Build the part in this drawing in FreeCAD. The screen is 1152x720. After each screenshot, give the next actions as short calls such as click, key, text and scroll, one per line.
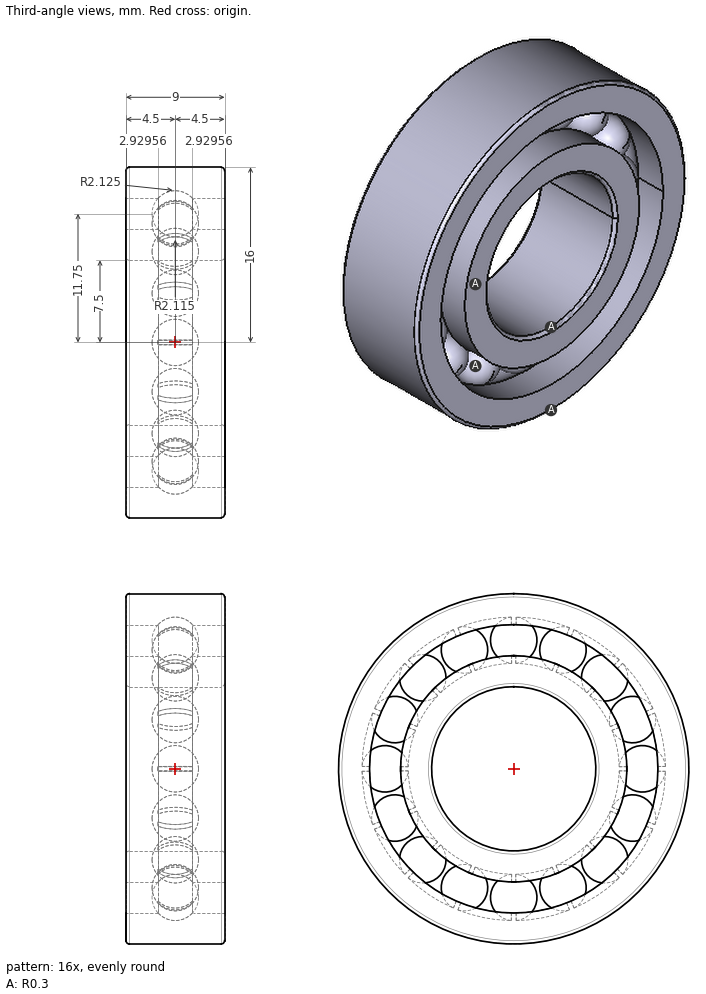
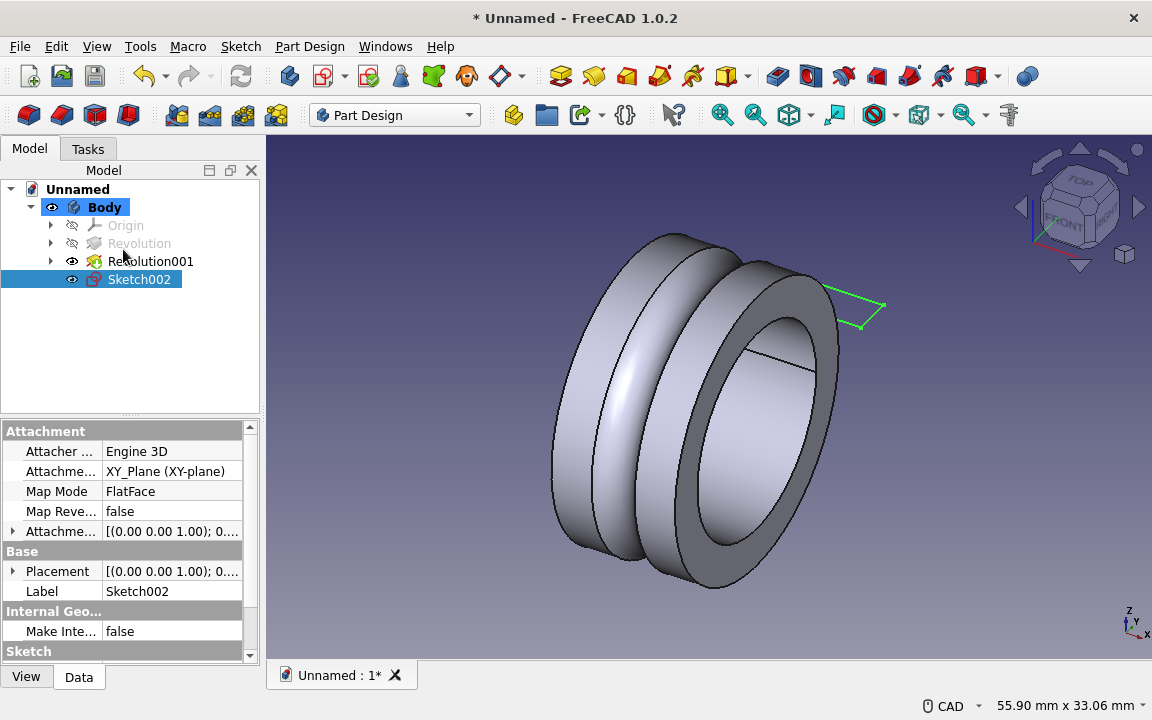
click(594, 76)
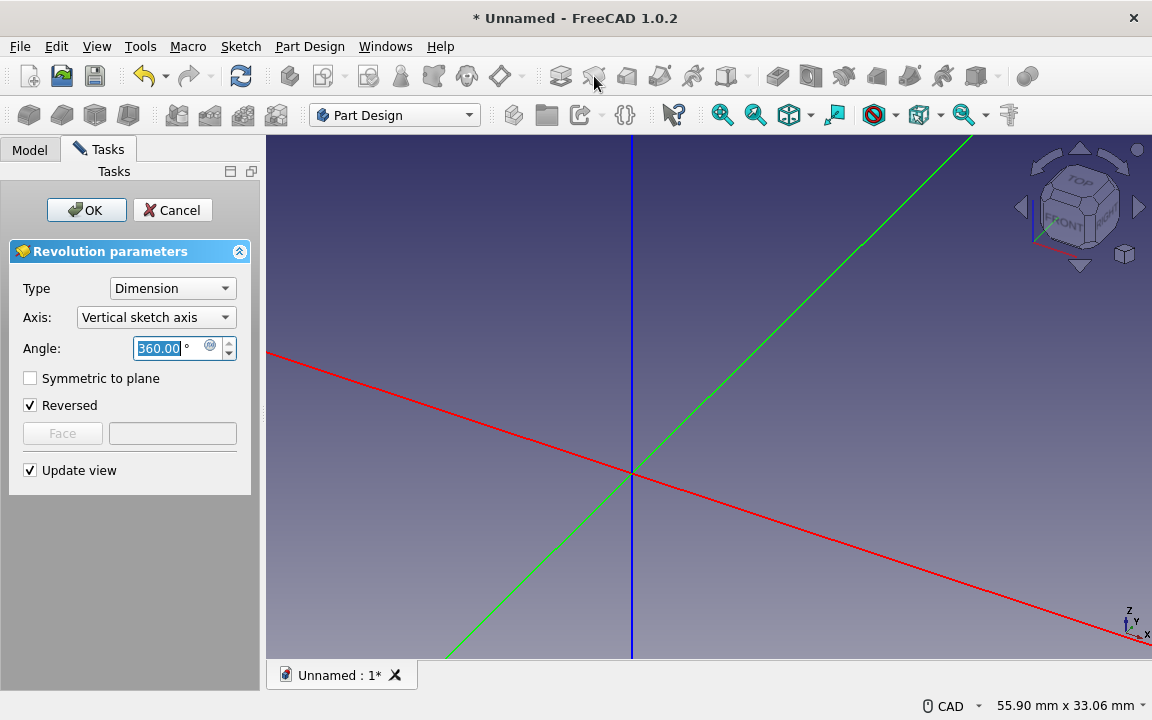
click(157, 318)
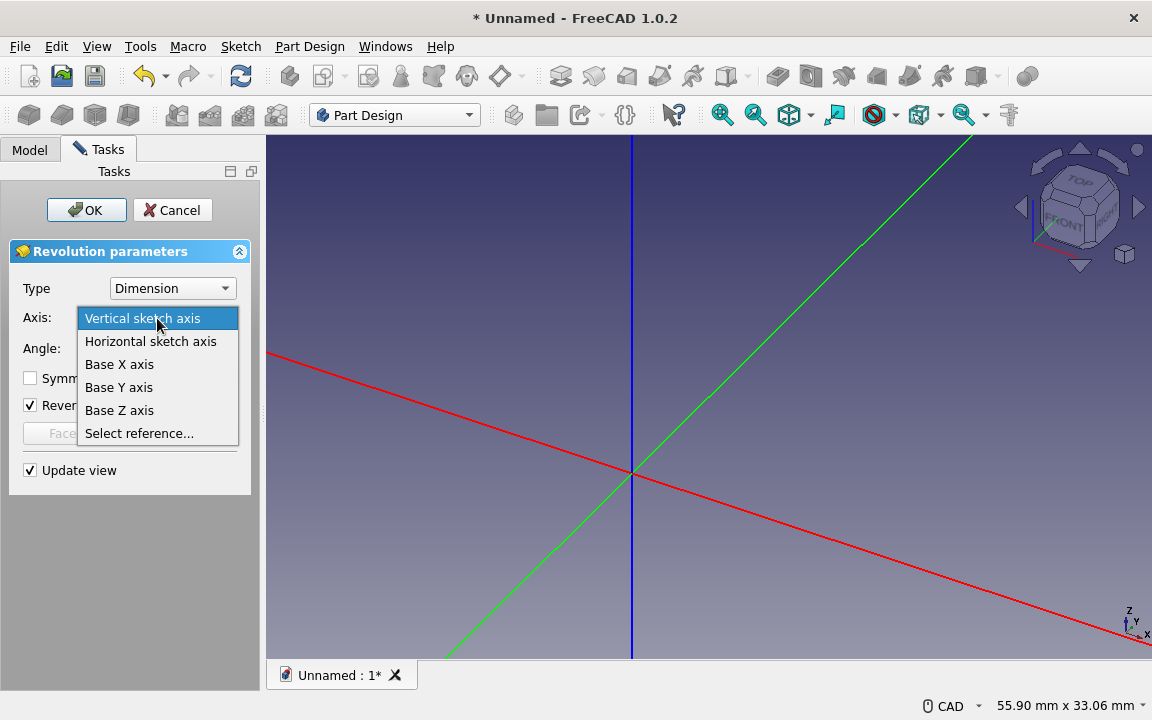
click(156, 342)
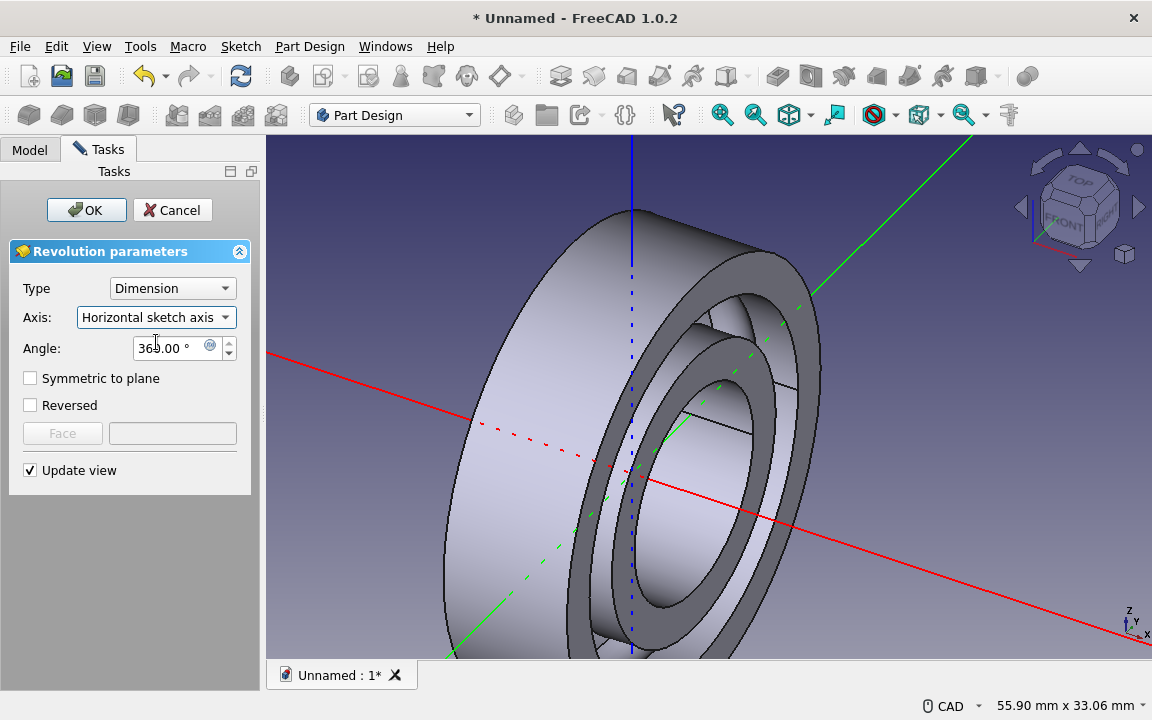
click(87, 210)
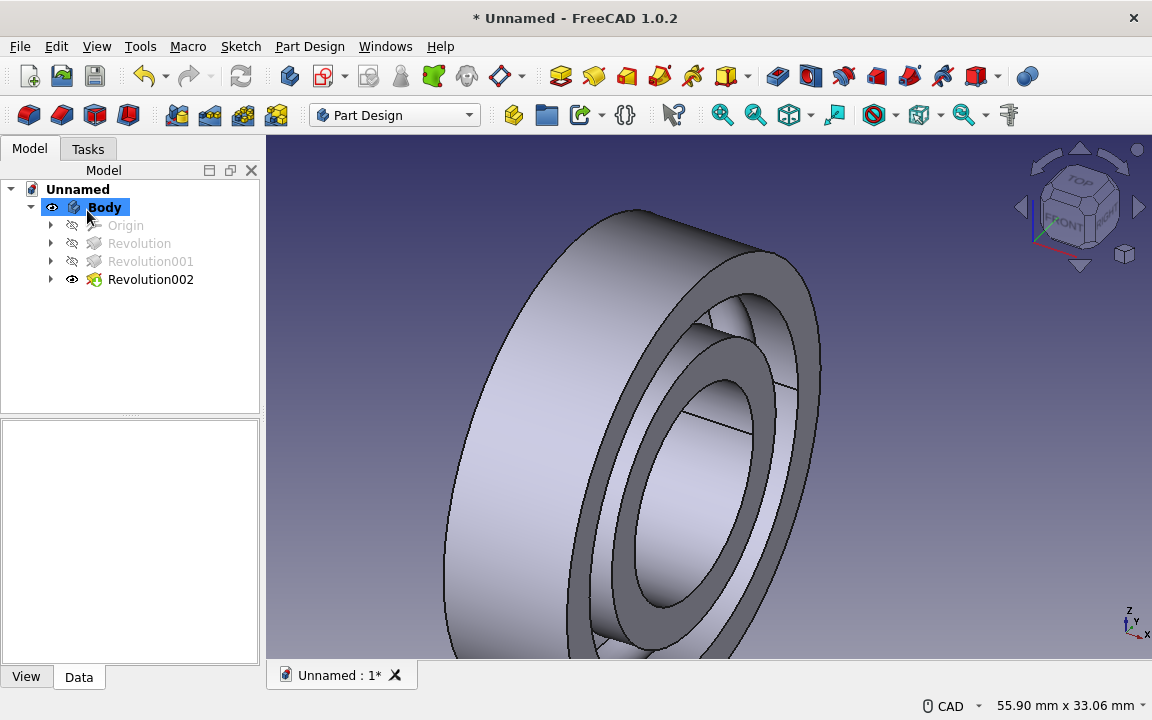
click(723, 116)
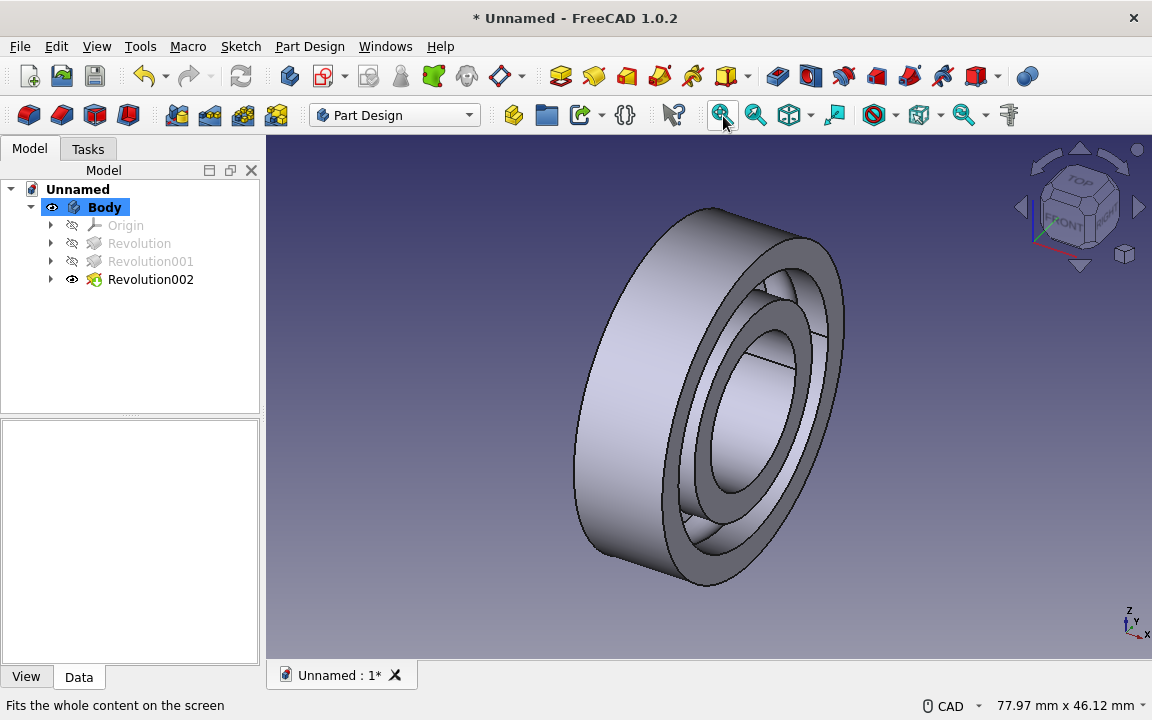
click(117, 243)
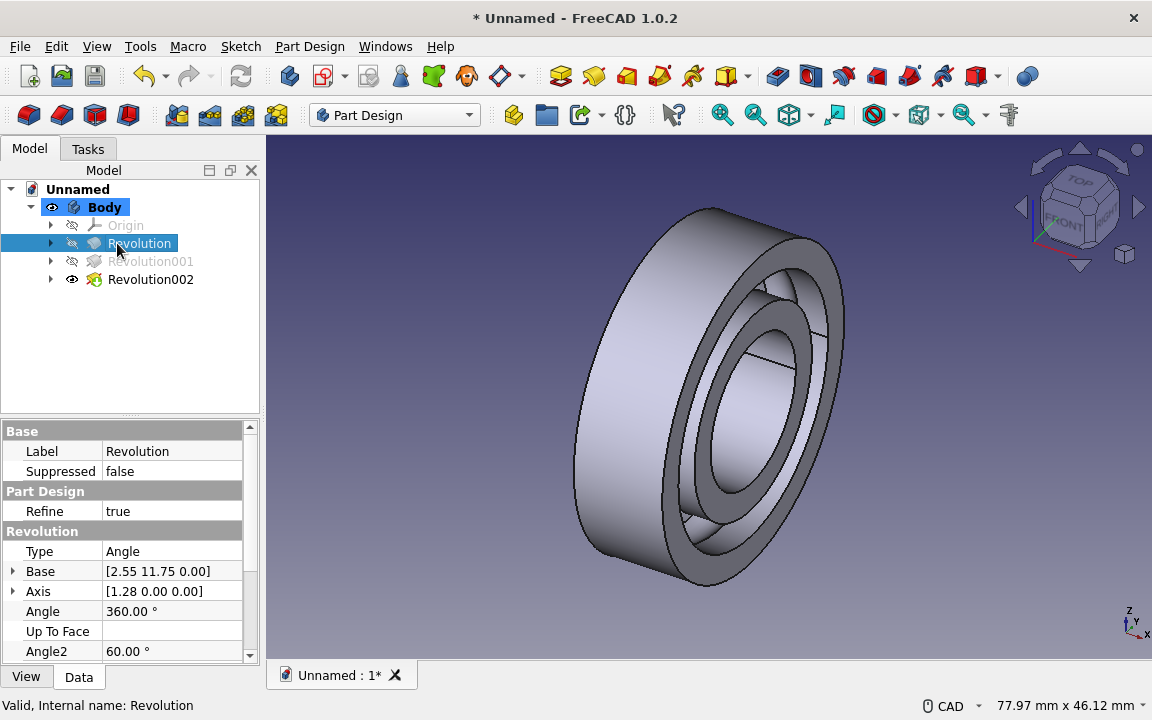
click(243, 116)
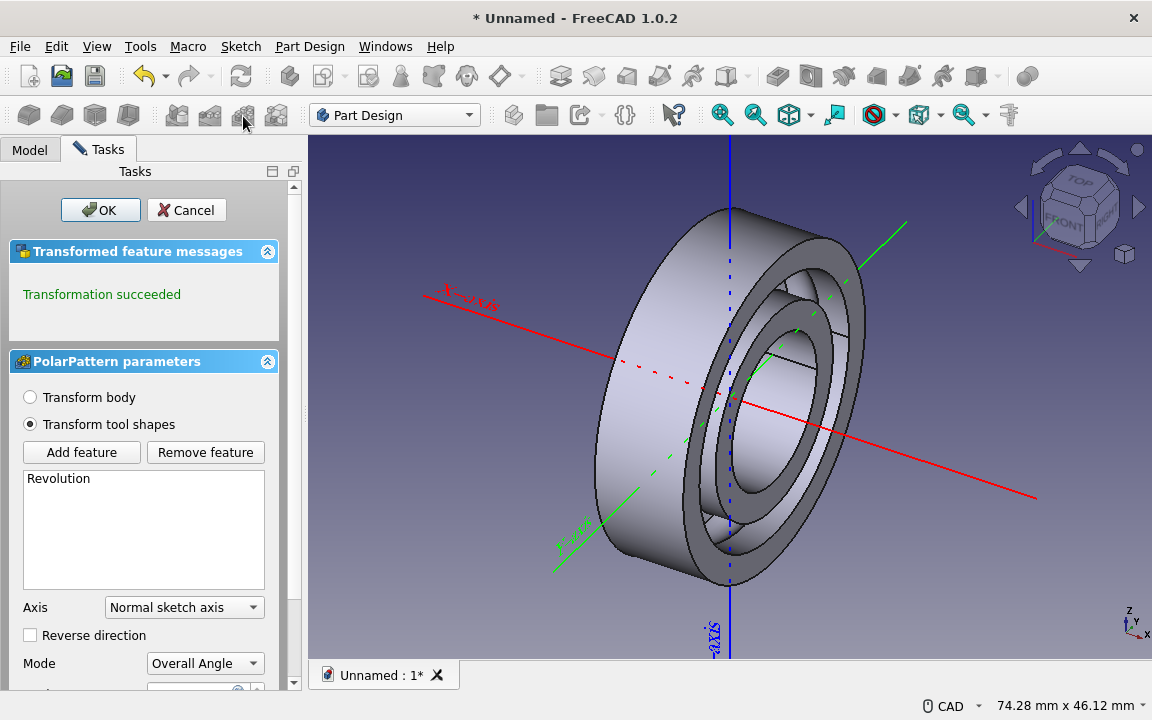
click(185, 608)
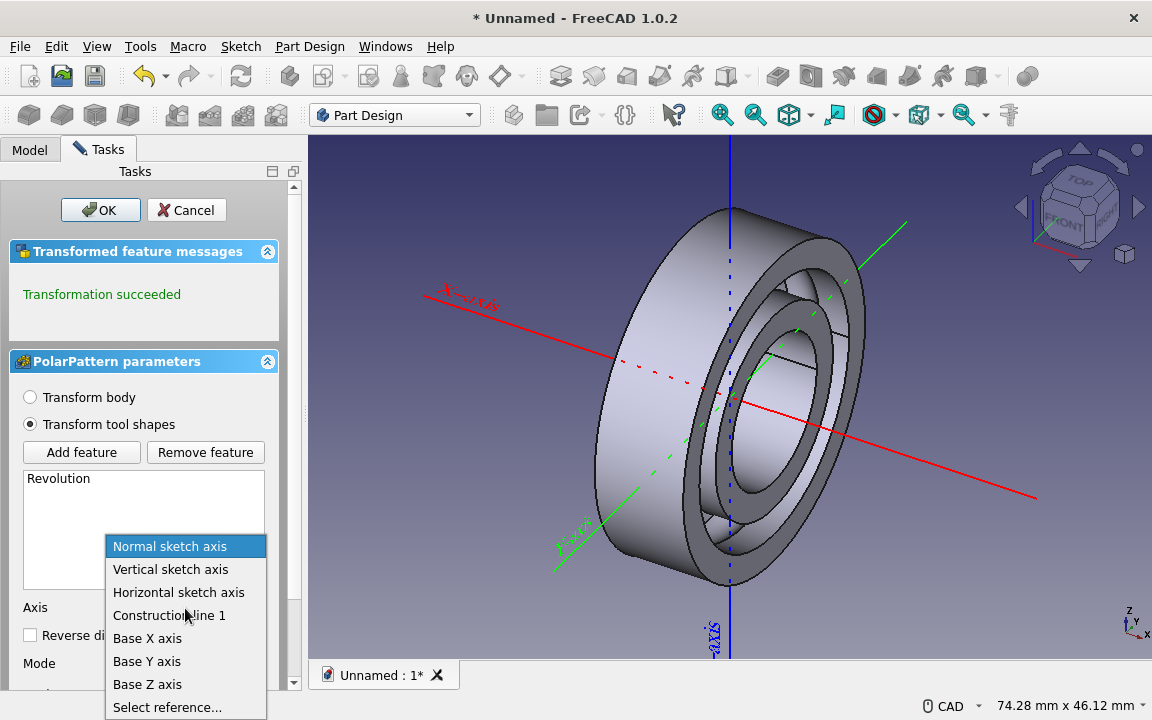
click(184, 638)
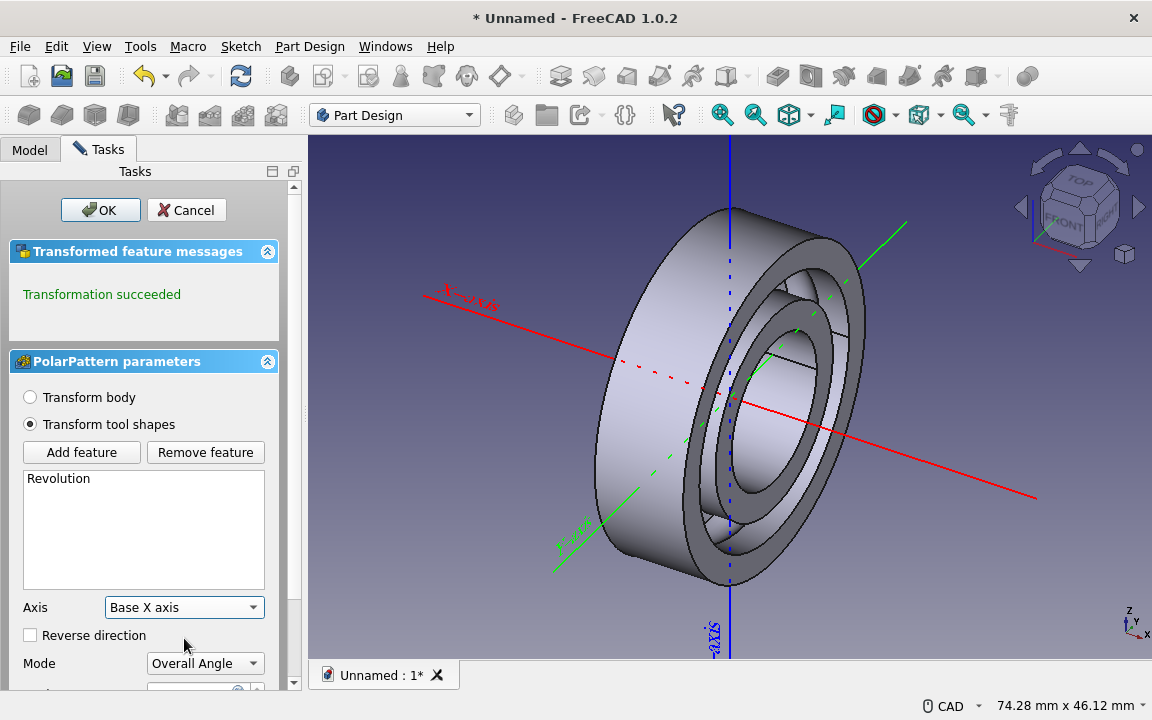
scroll(294, 436, down, 2)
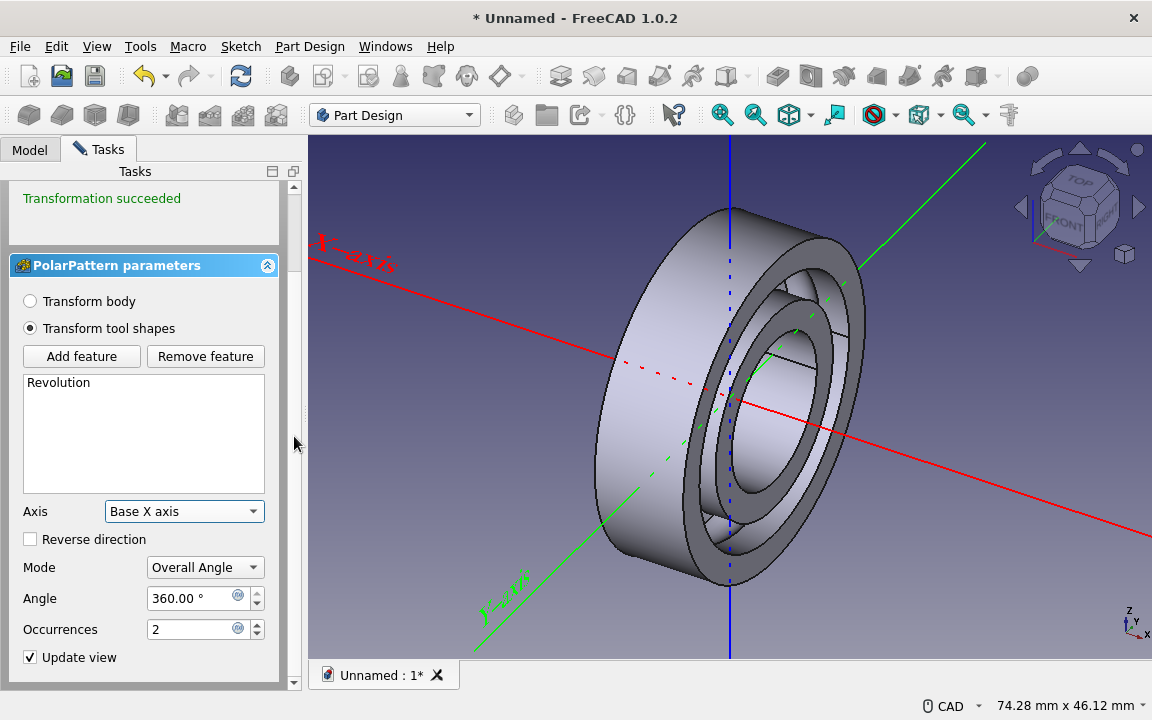
triple_click(199, 630)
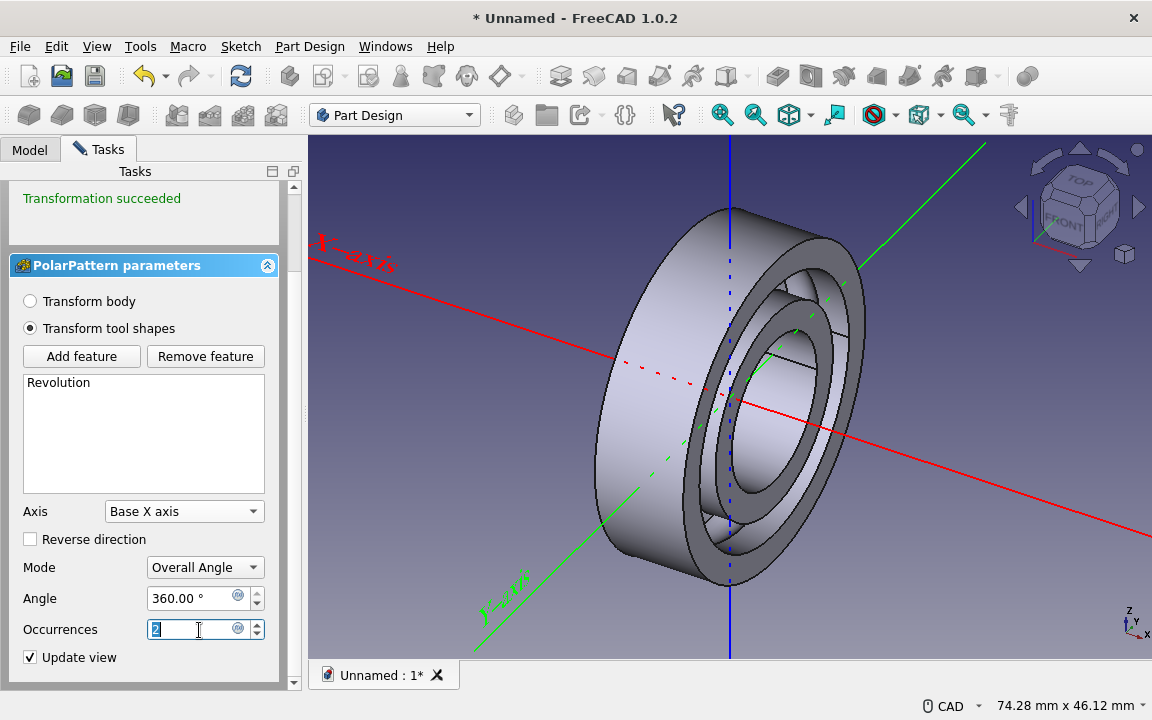
text(16)
key(Tab)